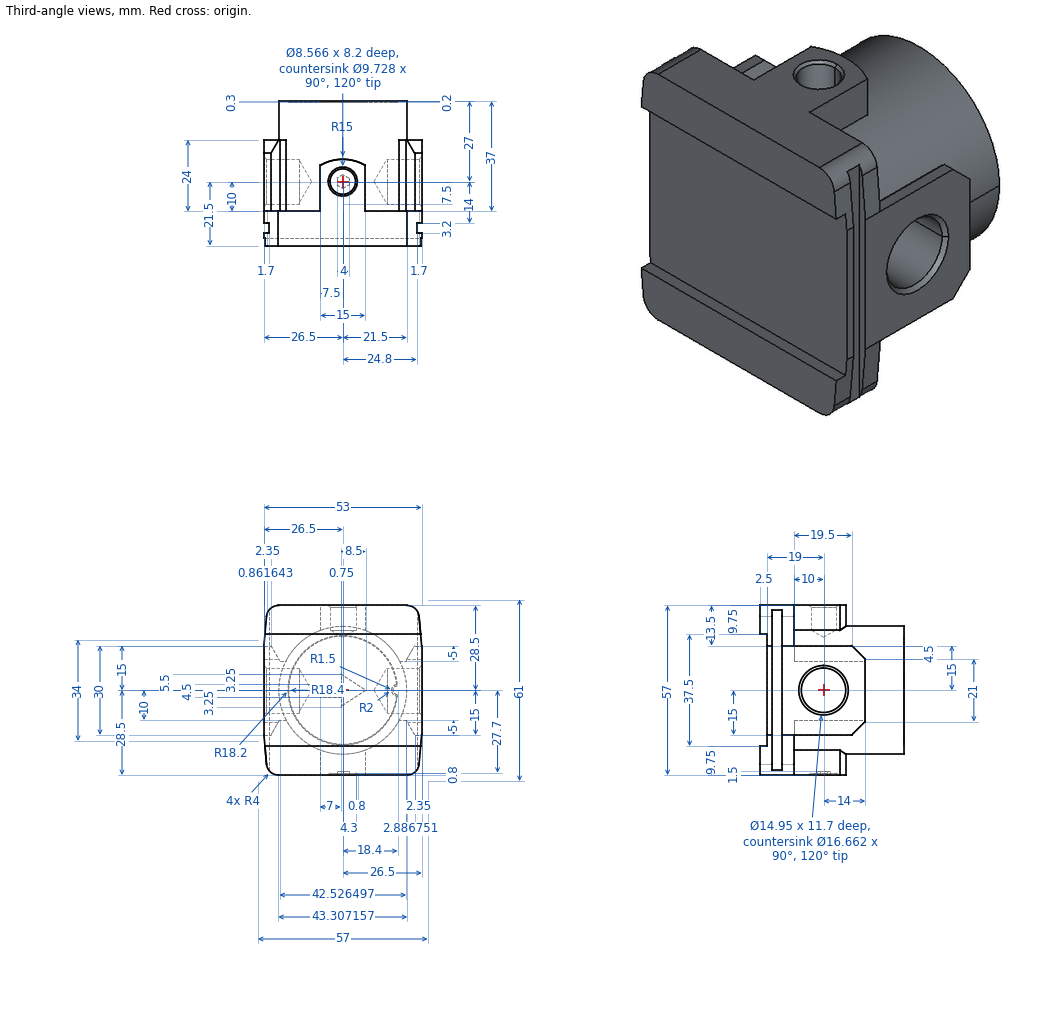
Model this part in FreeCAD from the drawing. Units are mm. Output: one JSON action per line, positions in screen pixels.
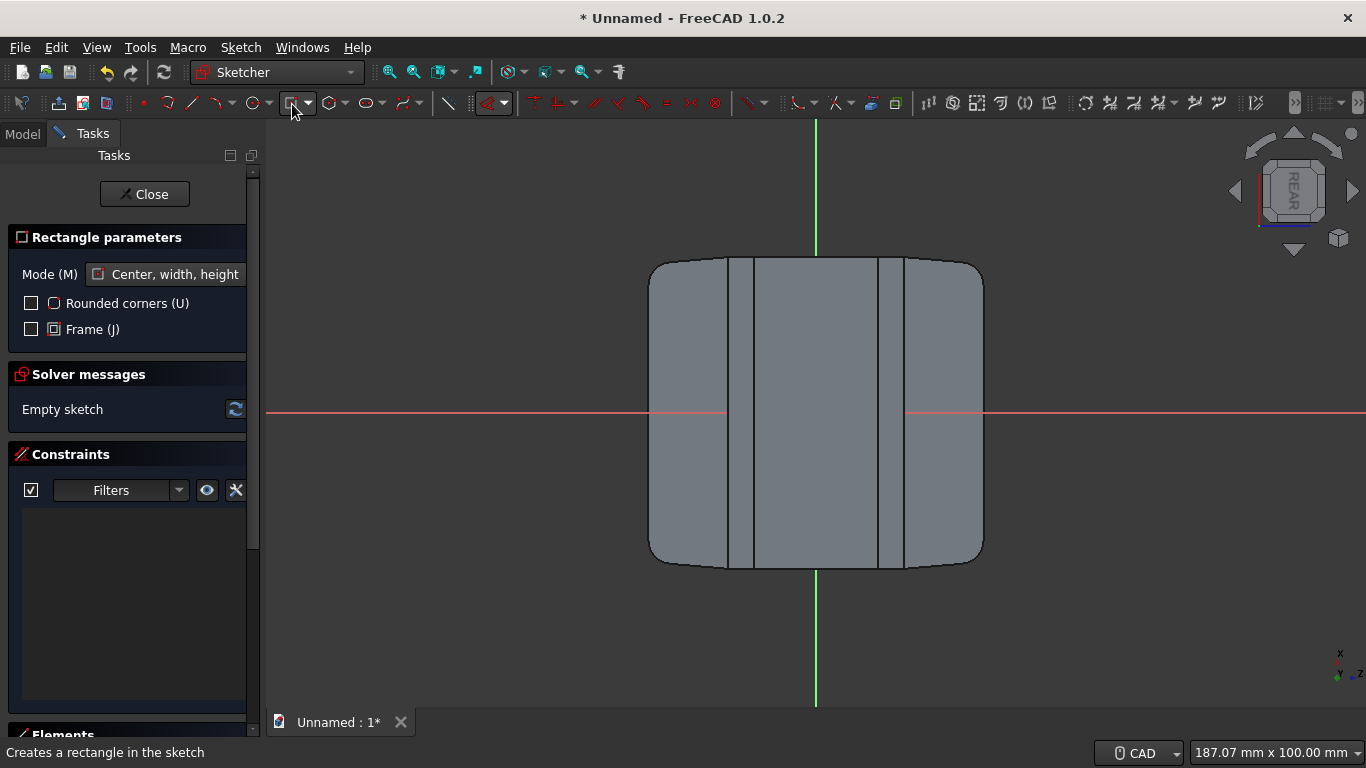
{"action": "left_click", "coordinate": [816, 413]}
{"action": "mouse_move", "coordinate": [916, 245]}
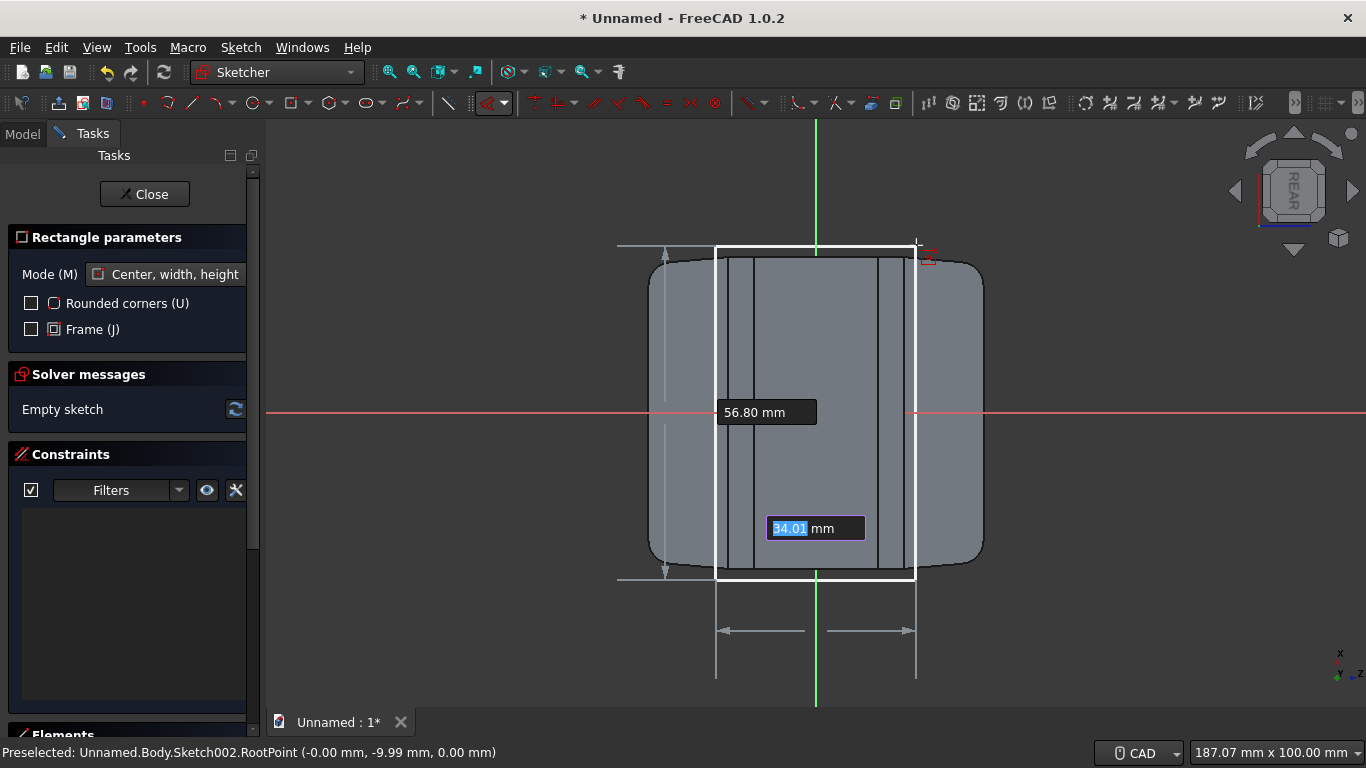
{"action": "type", "text": "34"}
{"action": "key", "text": "Tab"}
{"action": "type", "text": "57"}
{"action": "key", "text": "Return"}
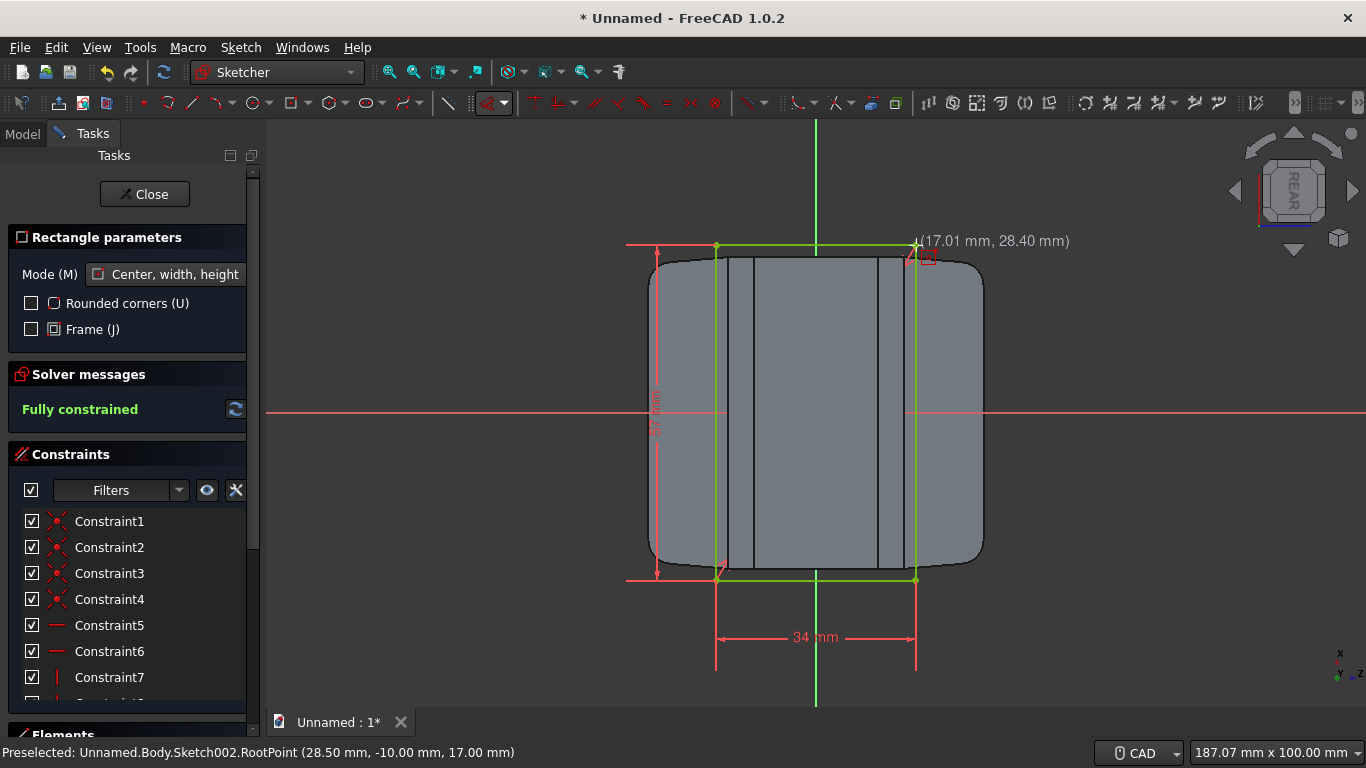
{"action": "key", "text": "g m"}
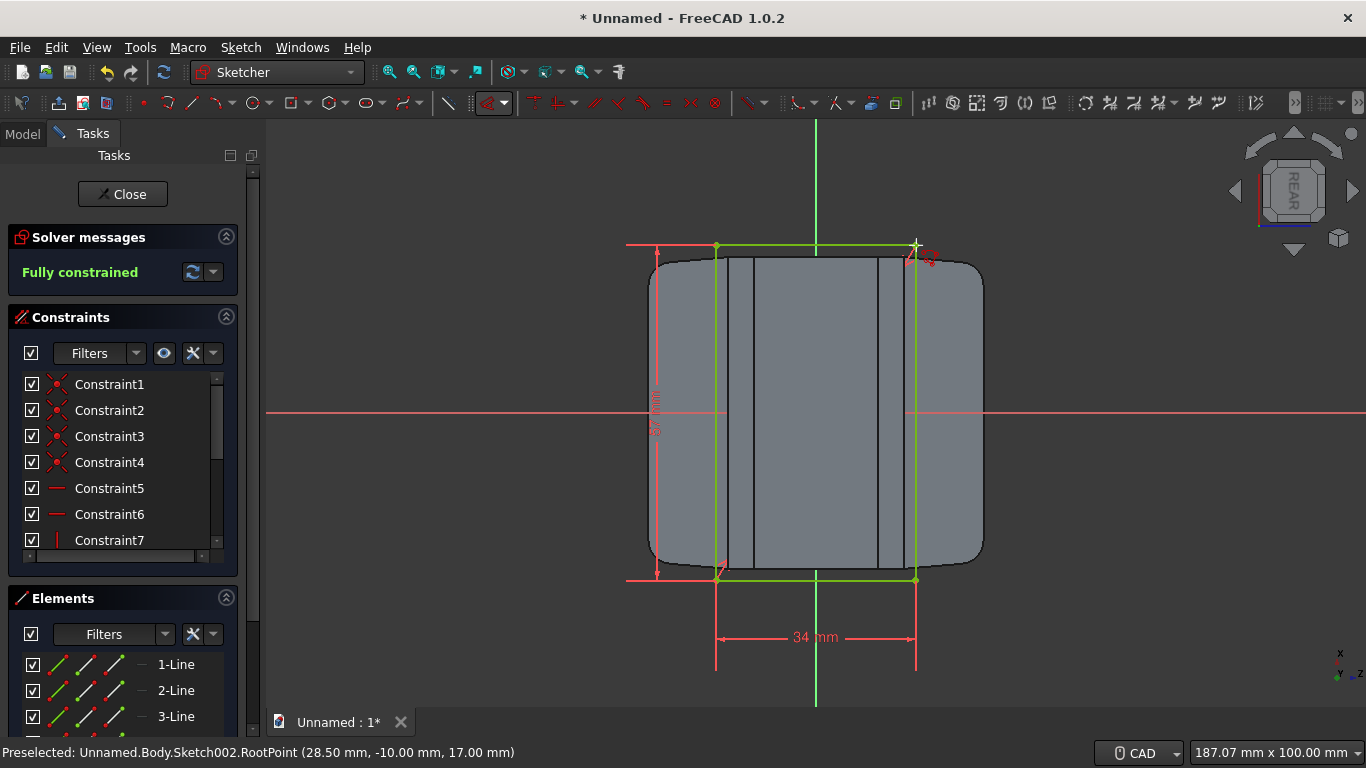
{"action": "left_click", "coordinate": [757, 538]}
{"action": "left_click", "coordinate": [757, 288]}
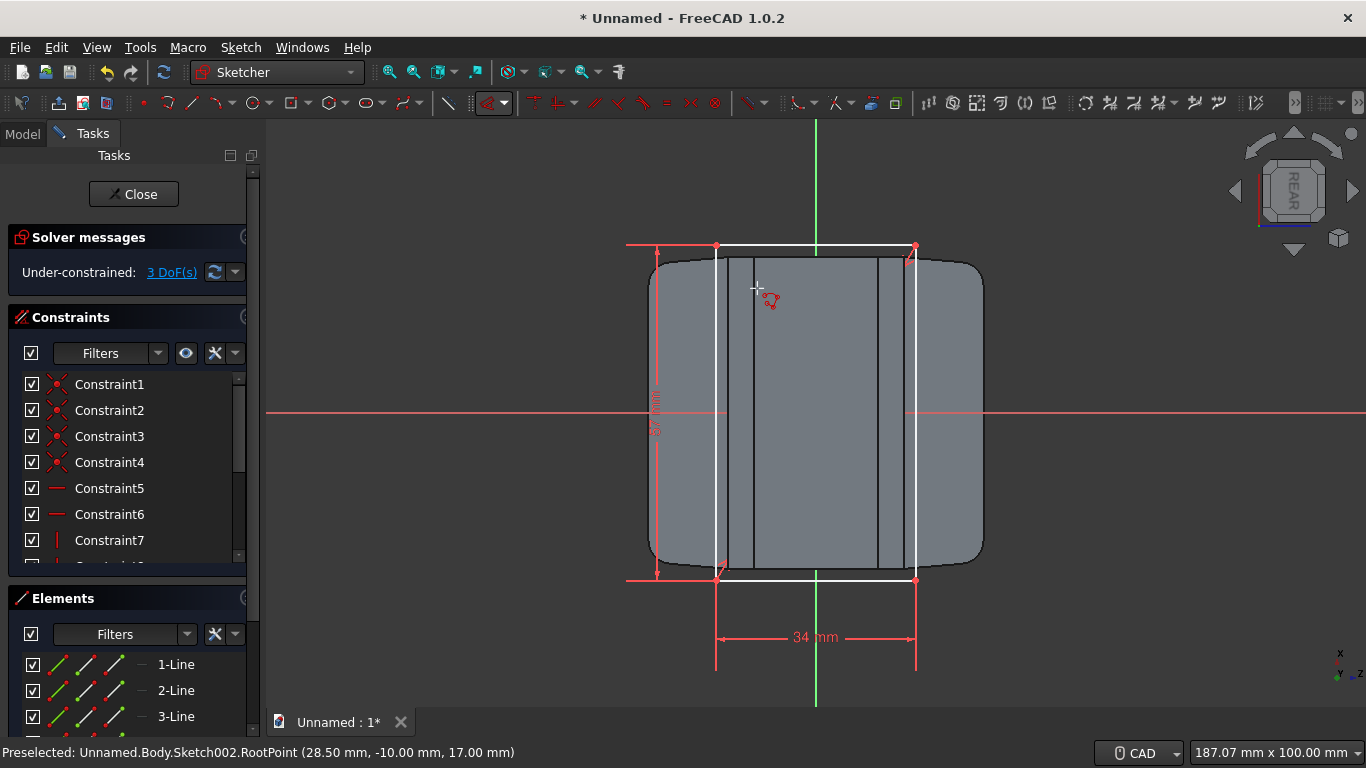
{"action": "scroll", "coordinate": [728, 271], "scroll_direction": "up", "scroll_amount": 2}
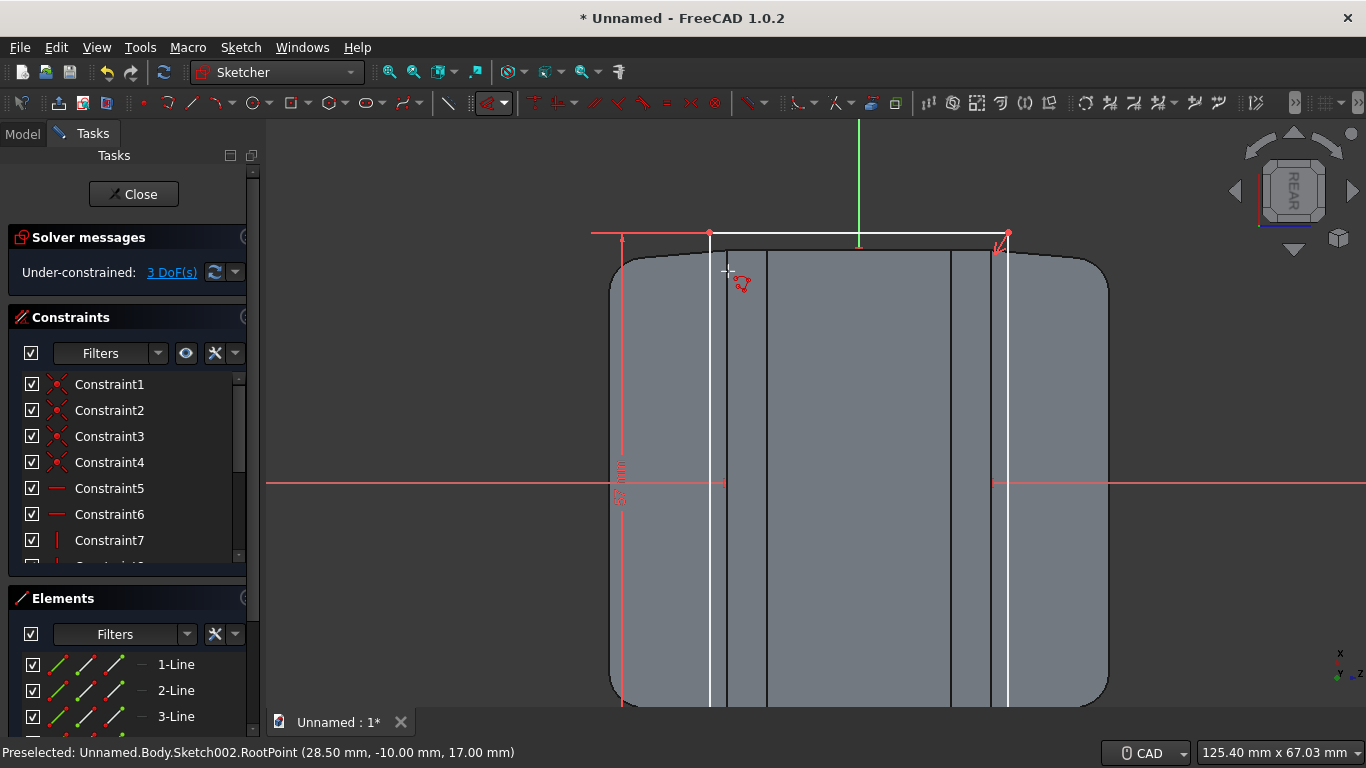
{"action": "left_click", "coordinate": [727, 271]}
{"action": "left_click", "coordinate": [727, 250]}
{"action": "left_click", "coordinate": [991, 250]}
{"action": "left_click", "coordinate": [991, 271]}
{"action": "left_click", "coordinate": [947, 296]}
{"action": "left_click", "coordinate": [947, 669]}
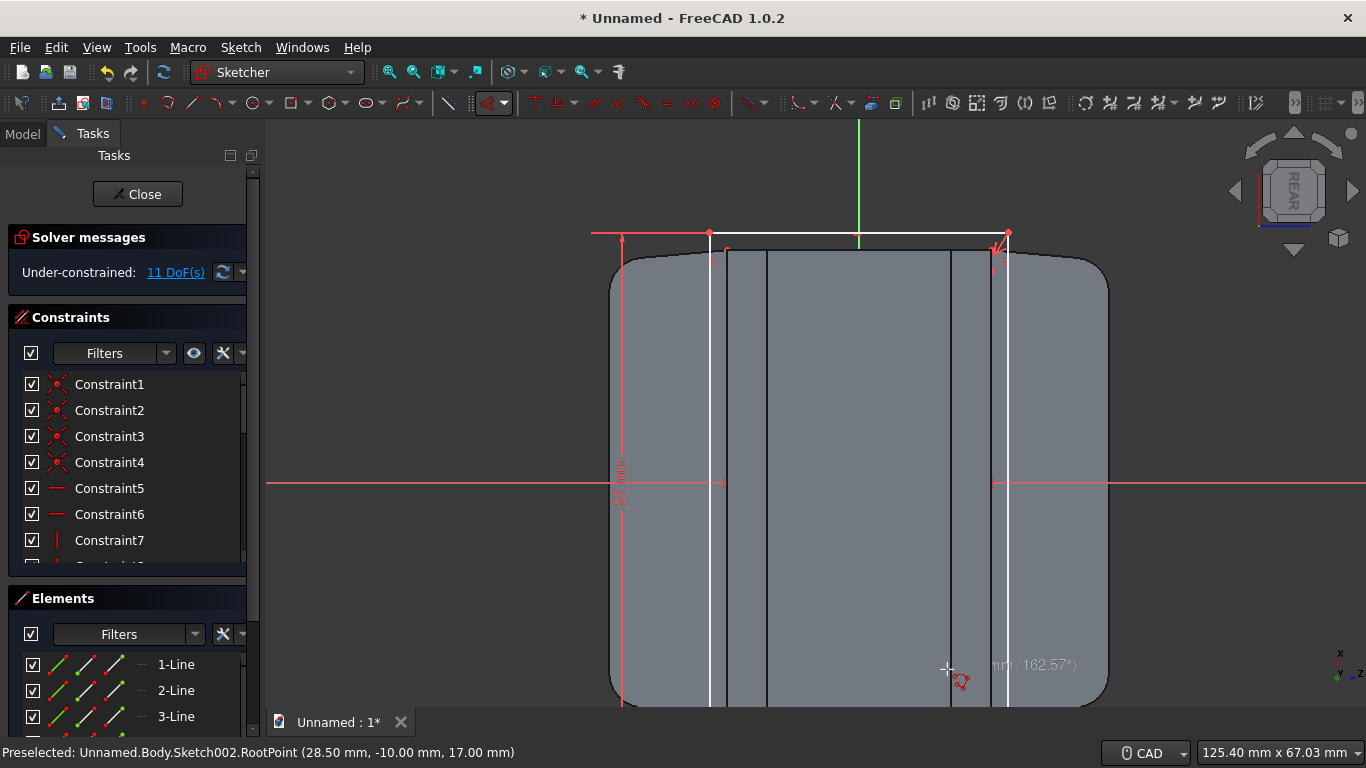
{"action": "scroll", "coordinate": [294, 147], "scroll_direction": "down", "scroll_amount": 1}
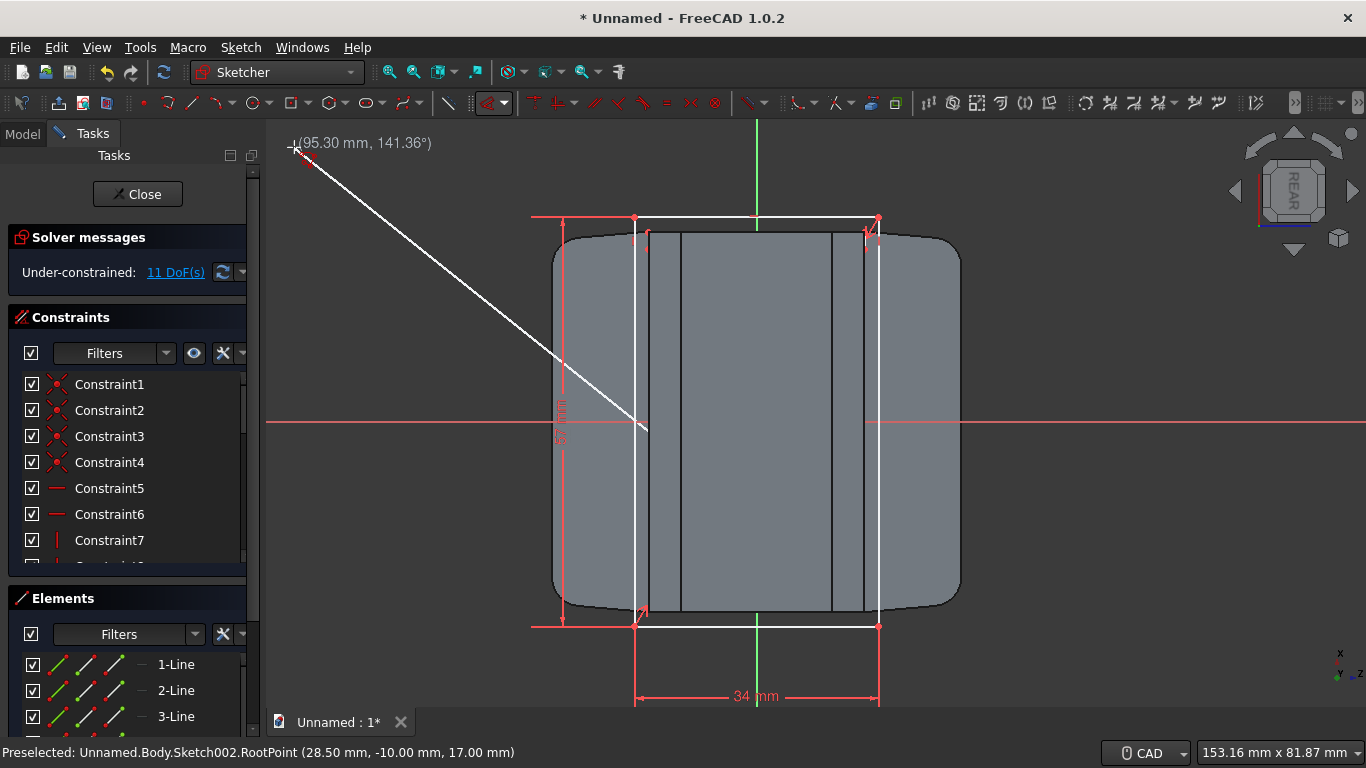
{"action": "left_click", "coordinate": [864, 595]}
{"action": "left_click", "coordinate": [864, 612]}
{"action": "left_click", "coordinate": [649, 612]}
{"action": "left_click", "coordinate": [649, 595]}
{"action": "left_click", "coordinate": [685, 576]}
{"action": "key", "text": "Escape"}
{"action": "key", "text": "Escape"}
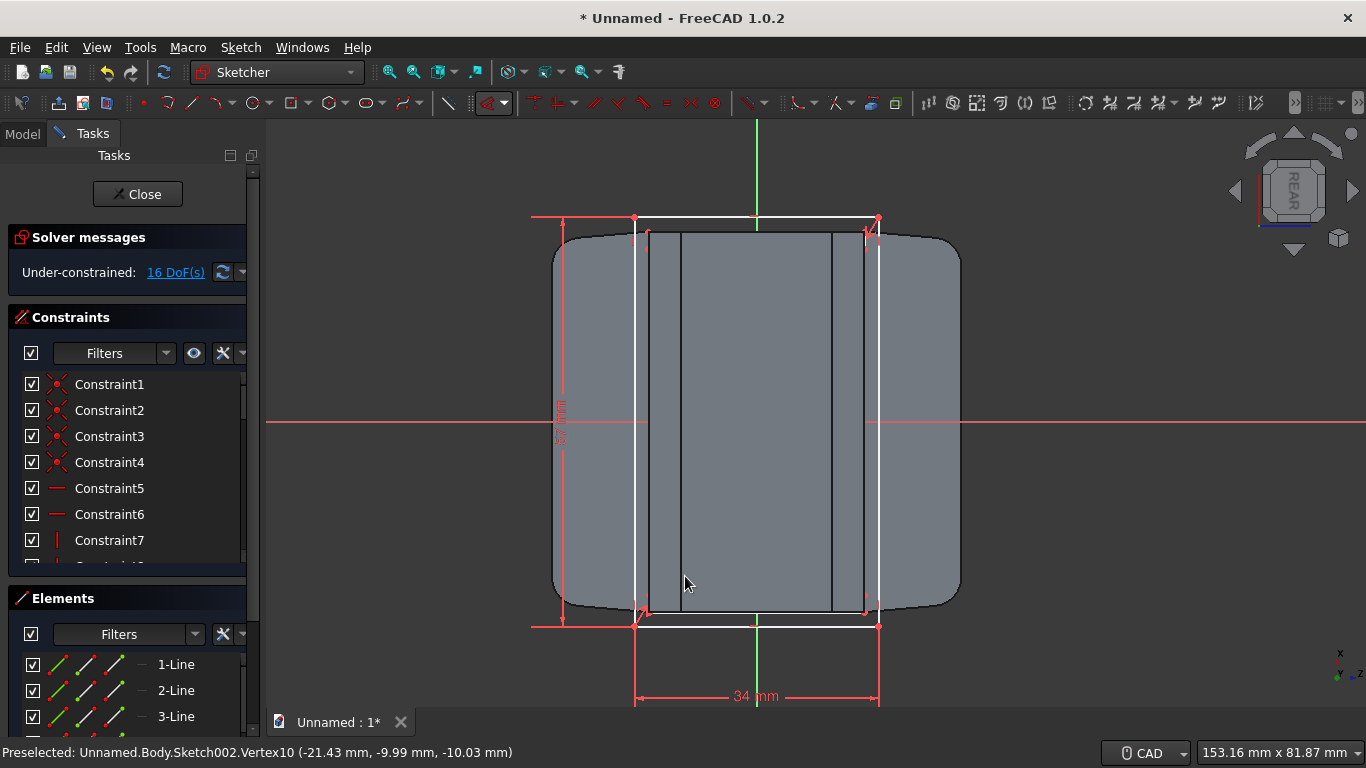
{"action": "left_click", "coordinate": [713, 232]}